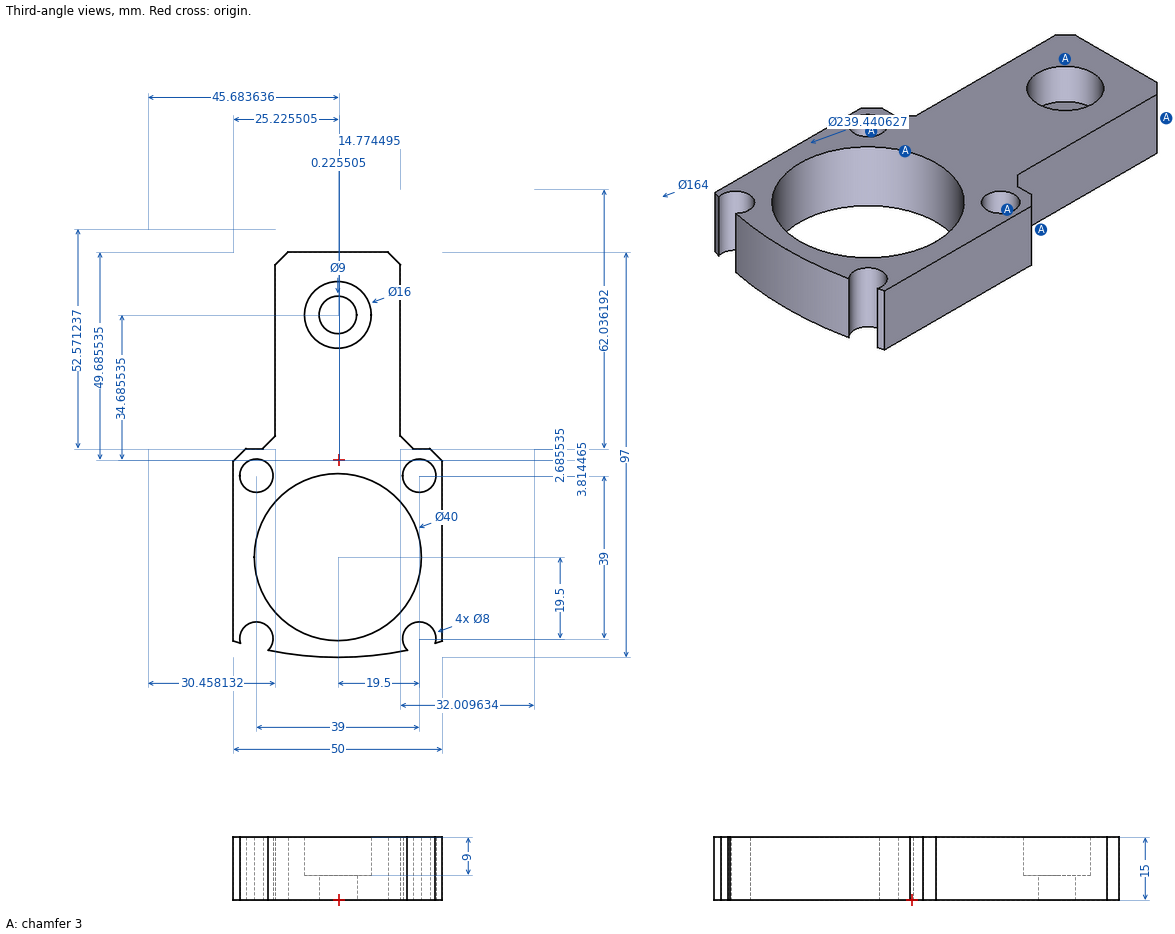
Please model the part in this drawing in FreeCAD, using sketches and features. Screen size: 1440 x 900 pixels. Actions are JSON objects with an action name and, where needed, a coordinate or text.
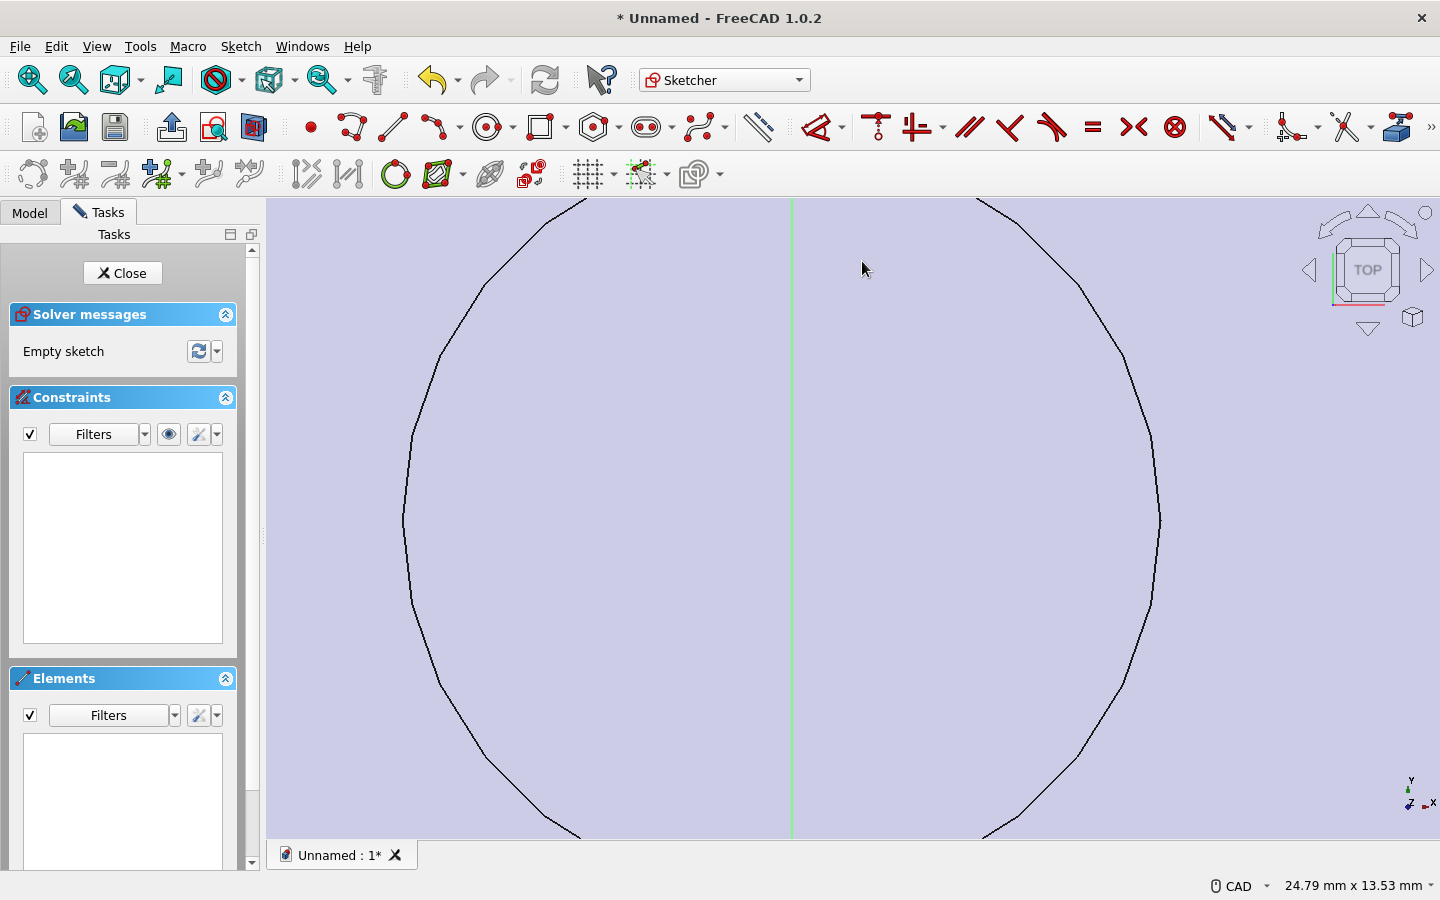
{"action": "key", "text": "g c"}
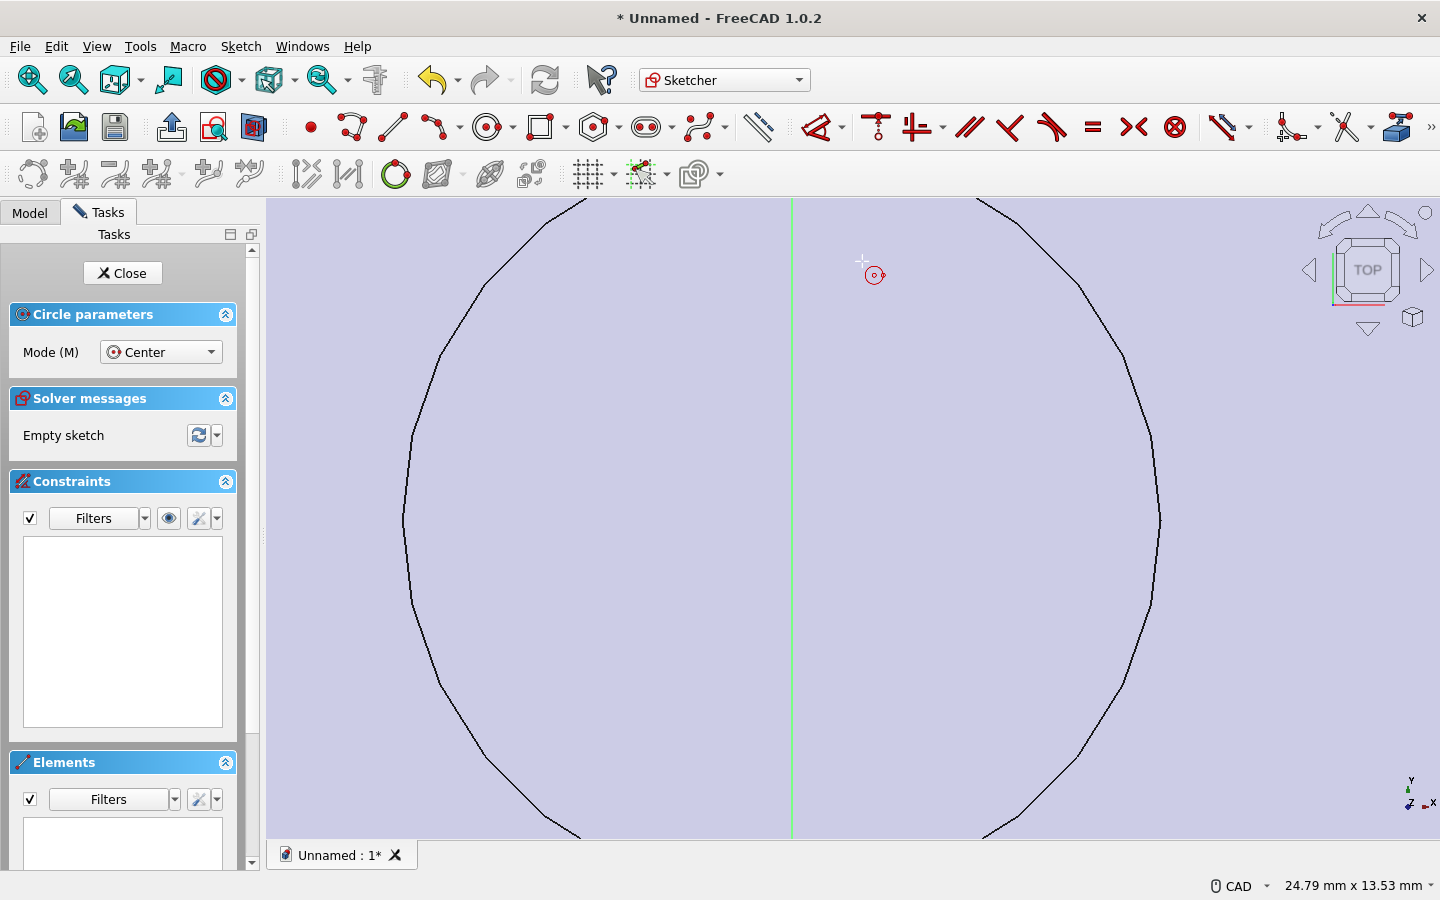
{"action": "scroll", "coordinate": [782, 520], "scroll_direction": "up", "scroll_amount": 2}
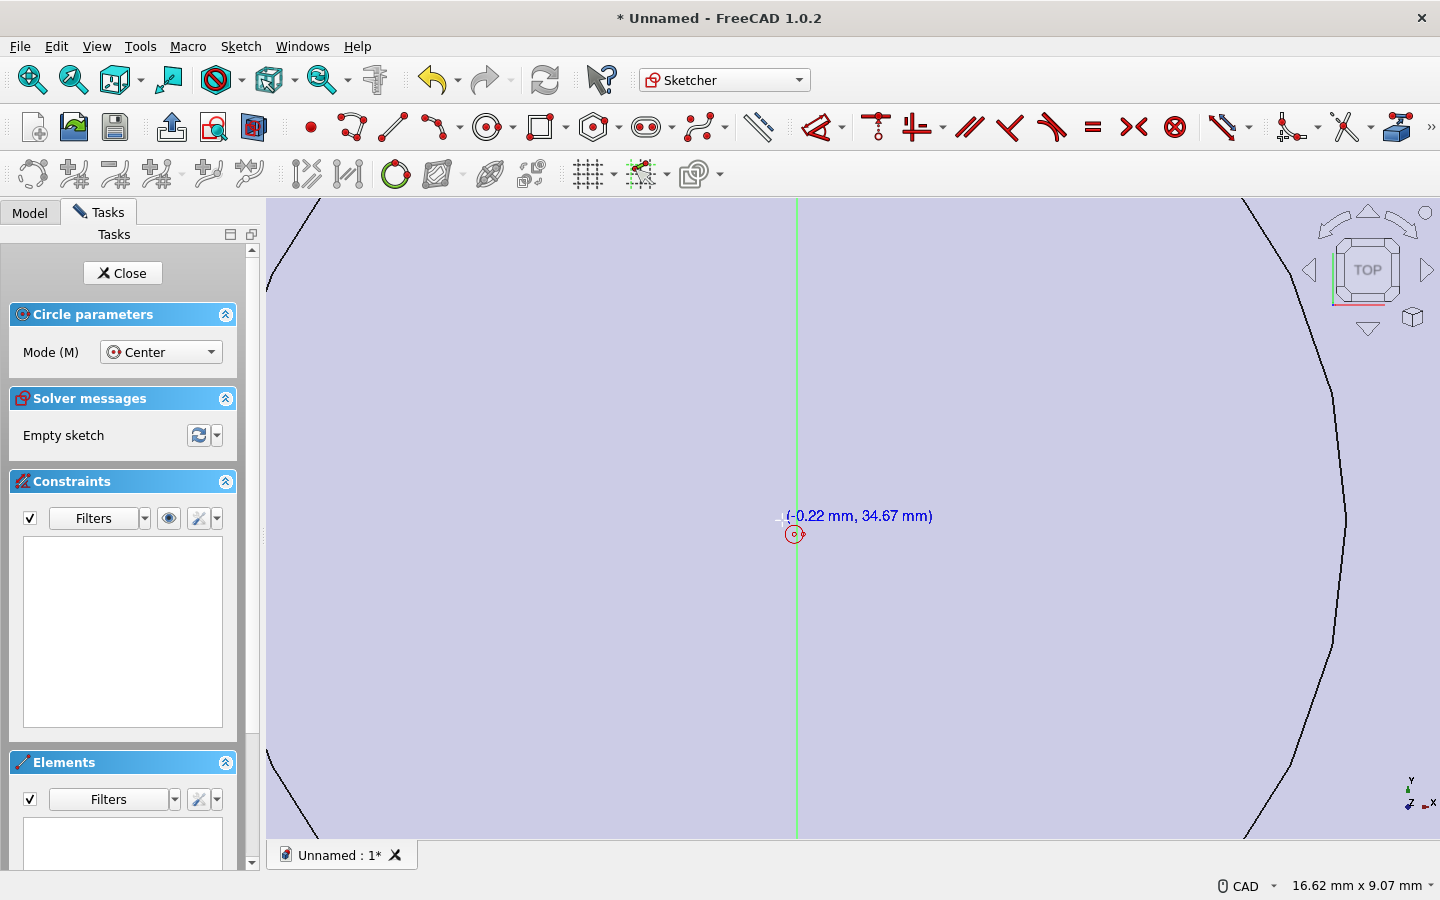
{"action": "left_click", "coordinate": [781, 520]}
{"action": "mouse_move", "coordinate": [1006, 295]}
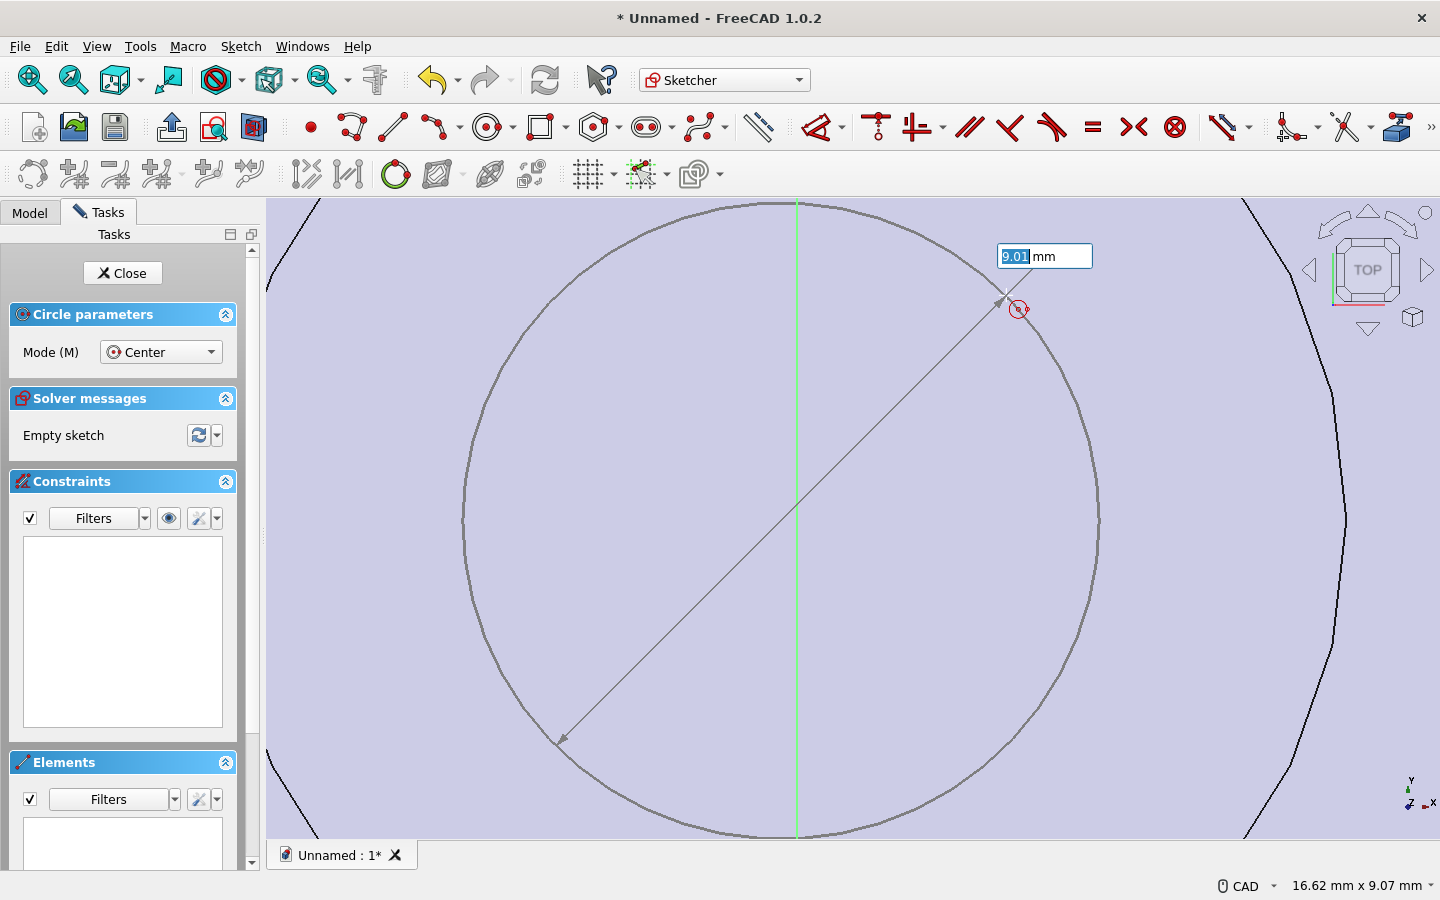
{"action": "type", "text": "9"}
{"action": "key", "text": "Return"}
{"action": "key", "text": "Escape"}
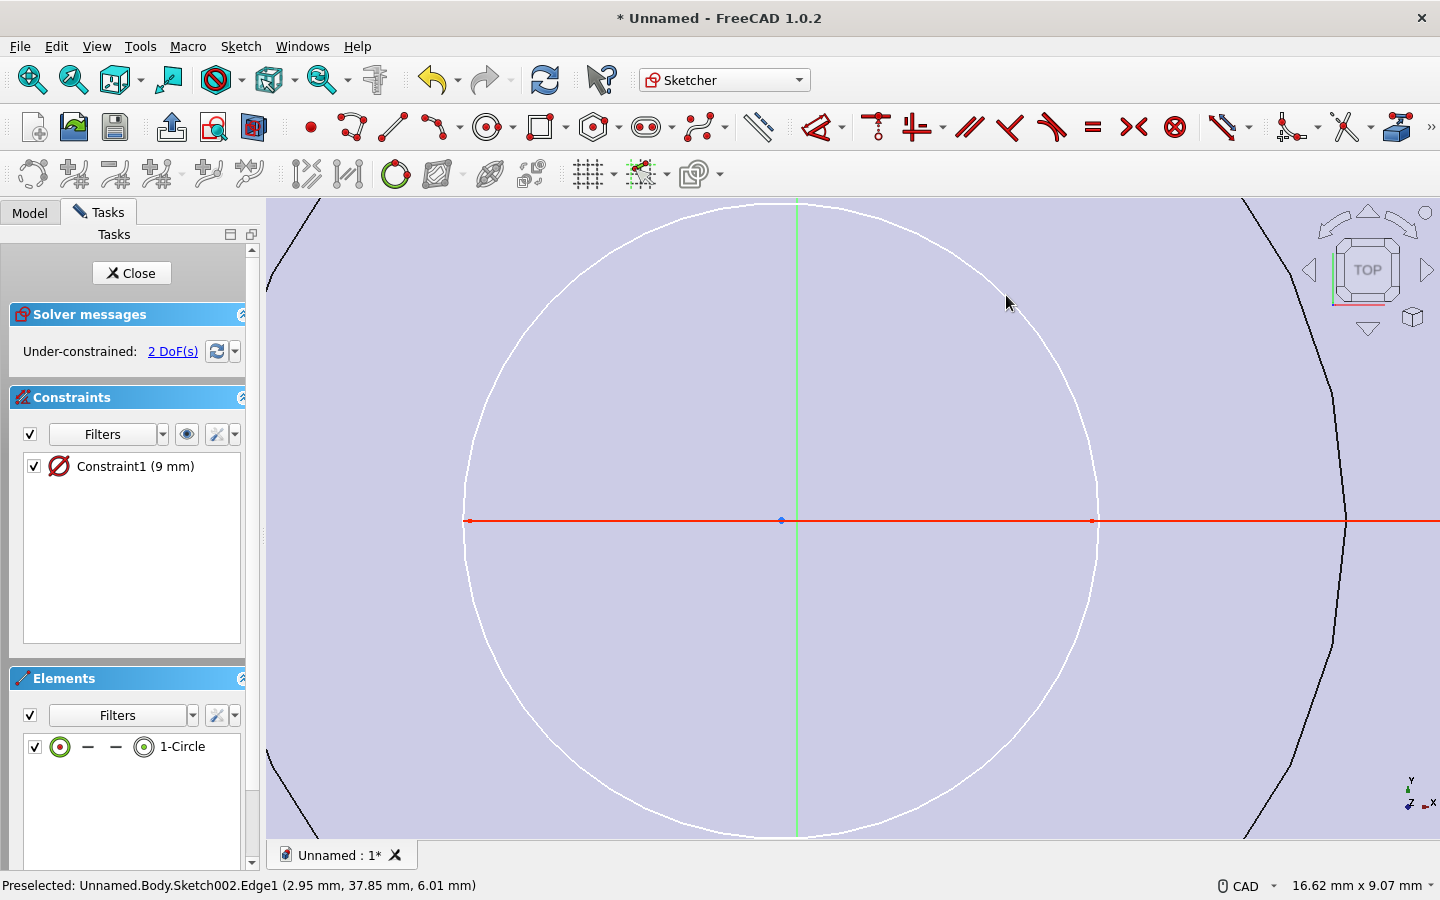
{"action": "key", "text": "d"}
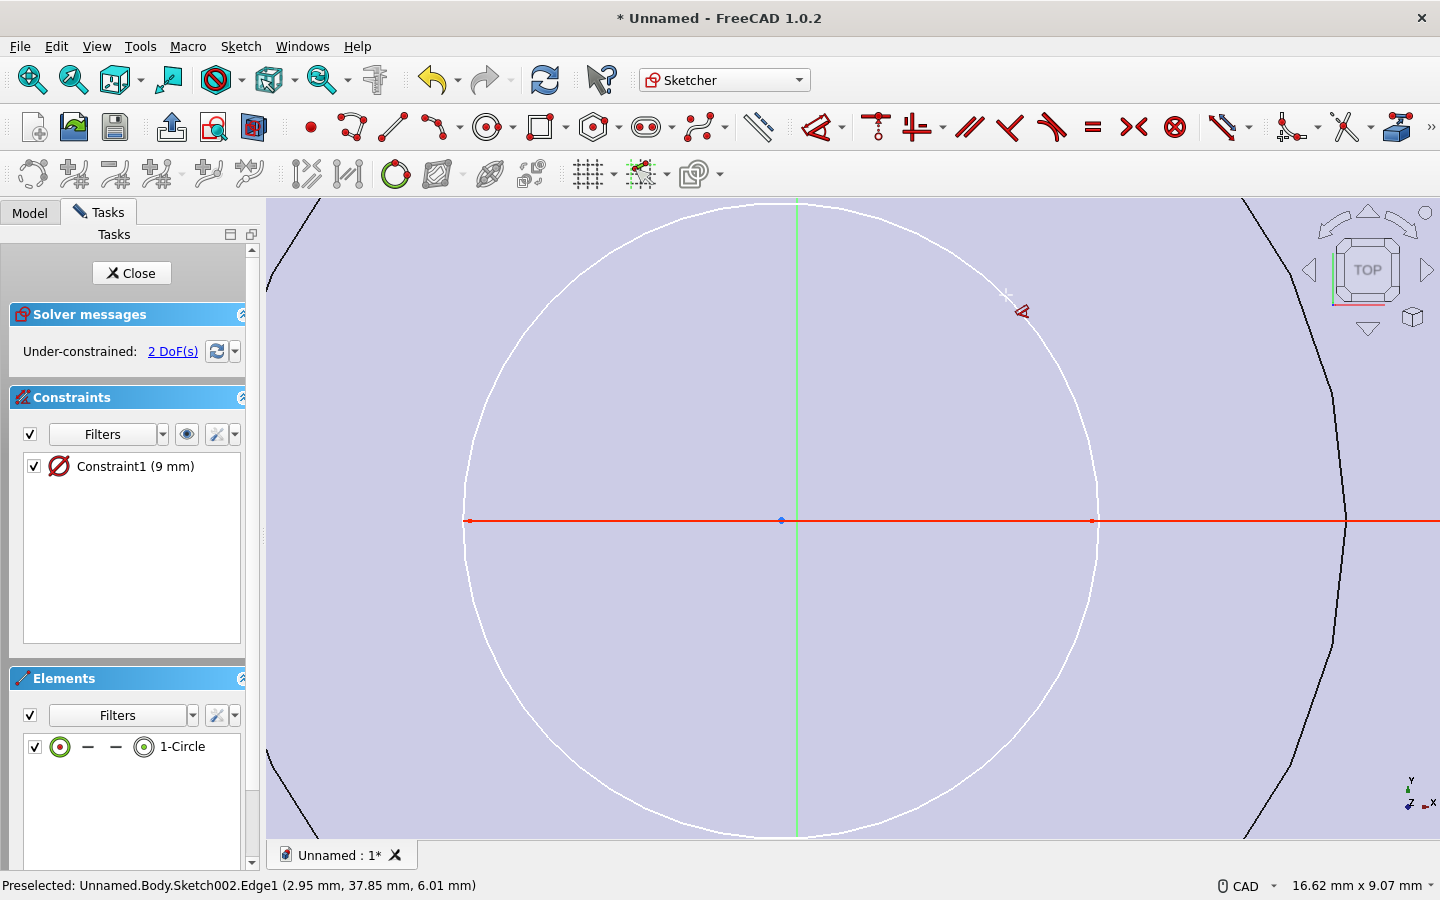
{"action": "scroll", "coordinate": [781, 521], "scroll_direction": "up", "scroll_amount": 5}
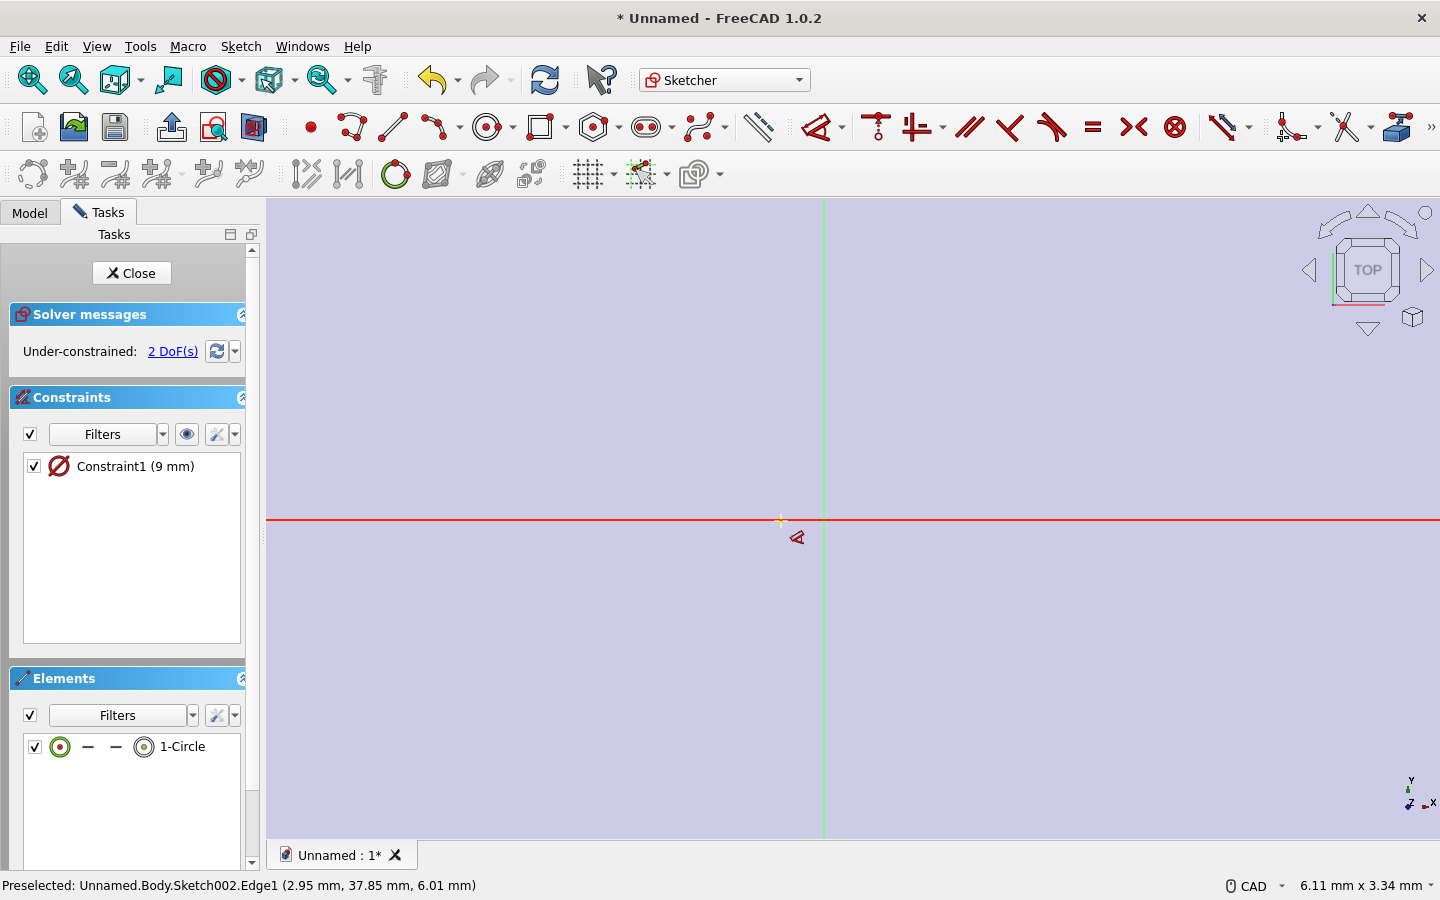
{"action": "left_click", "coordinate": [780, 520]}
{"action": "left_click", "coordinate": [802, 486]}